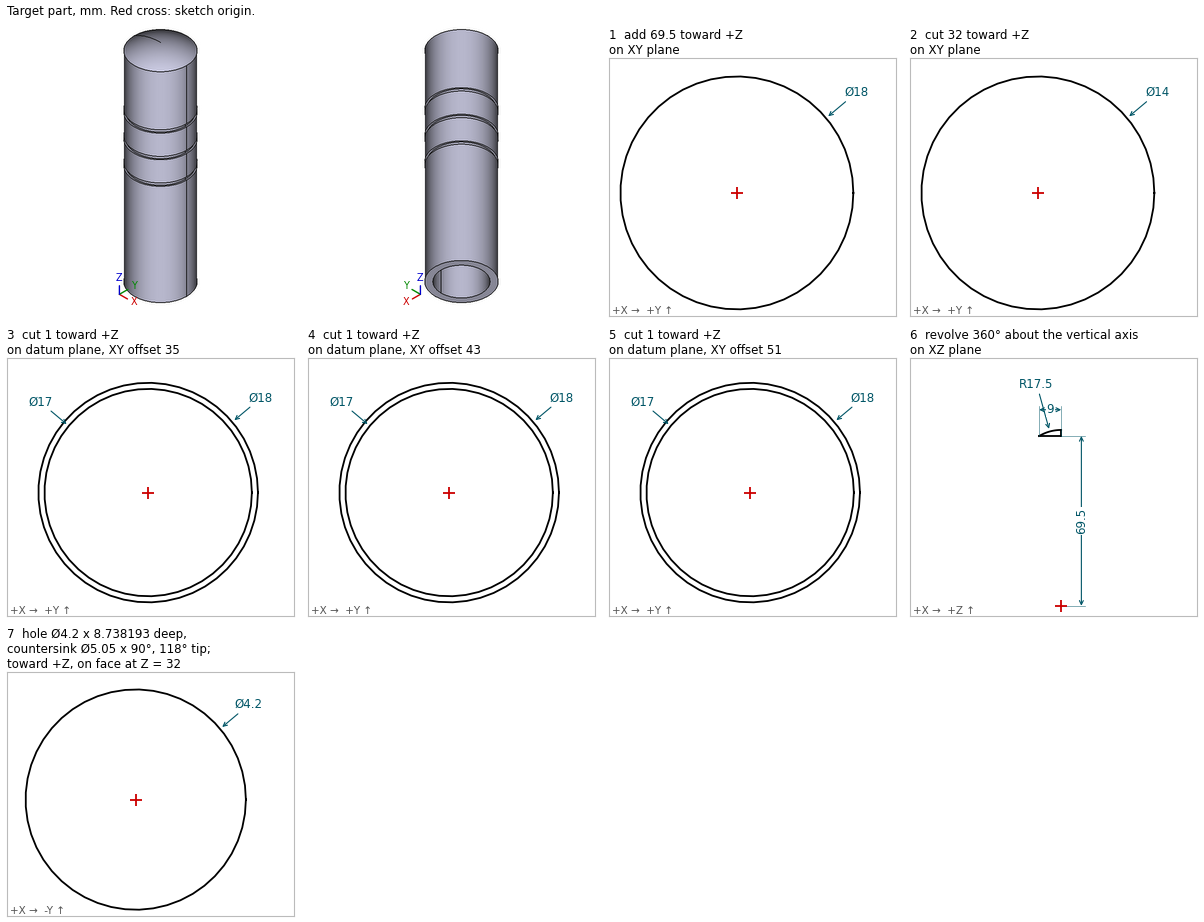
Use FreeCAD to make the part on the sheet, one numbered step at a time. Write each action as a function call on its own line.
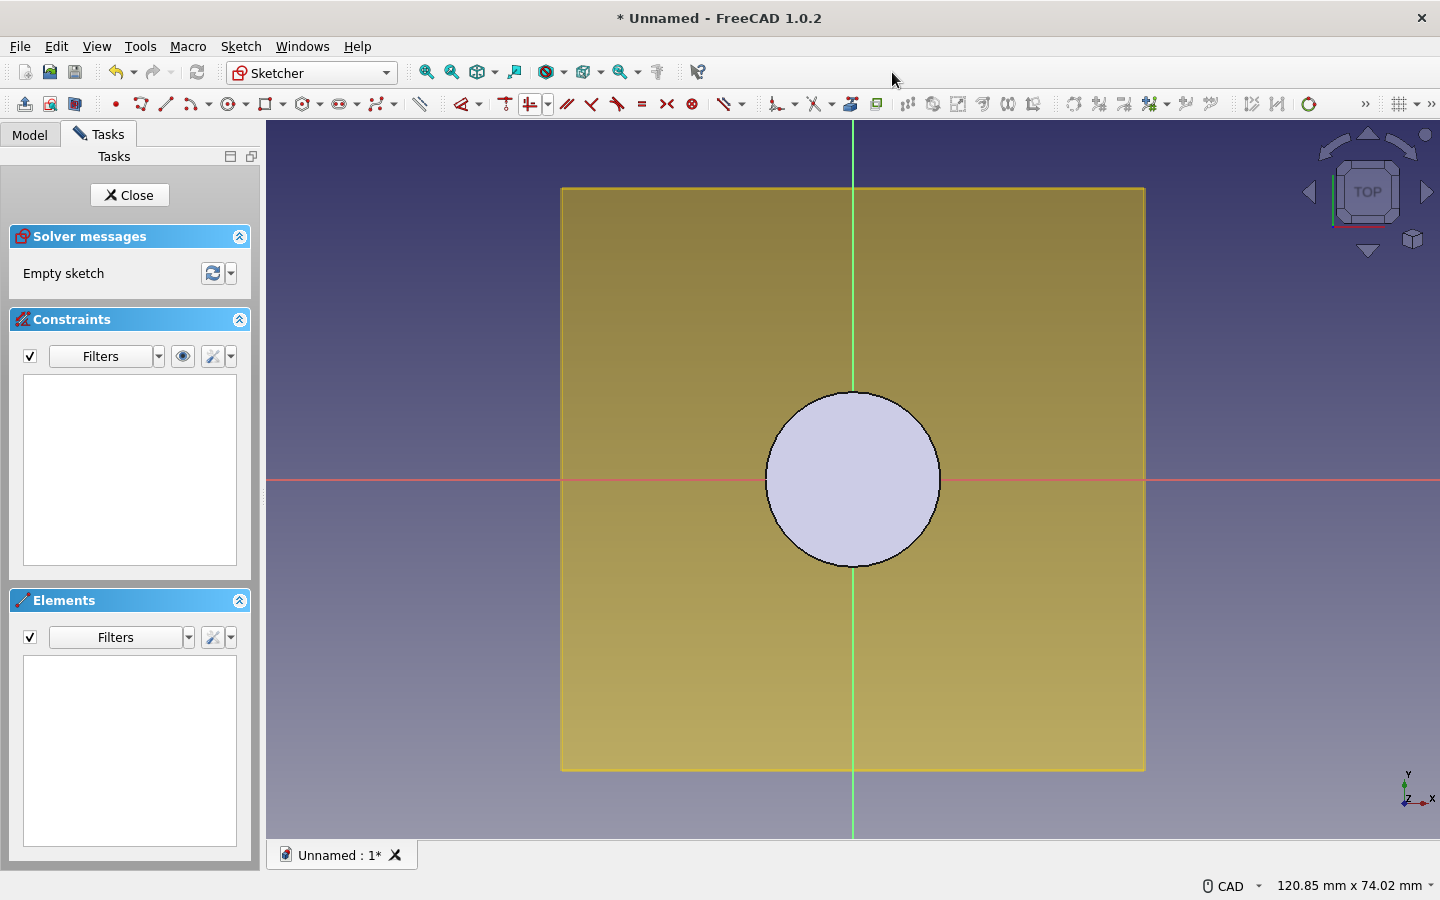
key(q)
key(s)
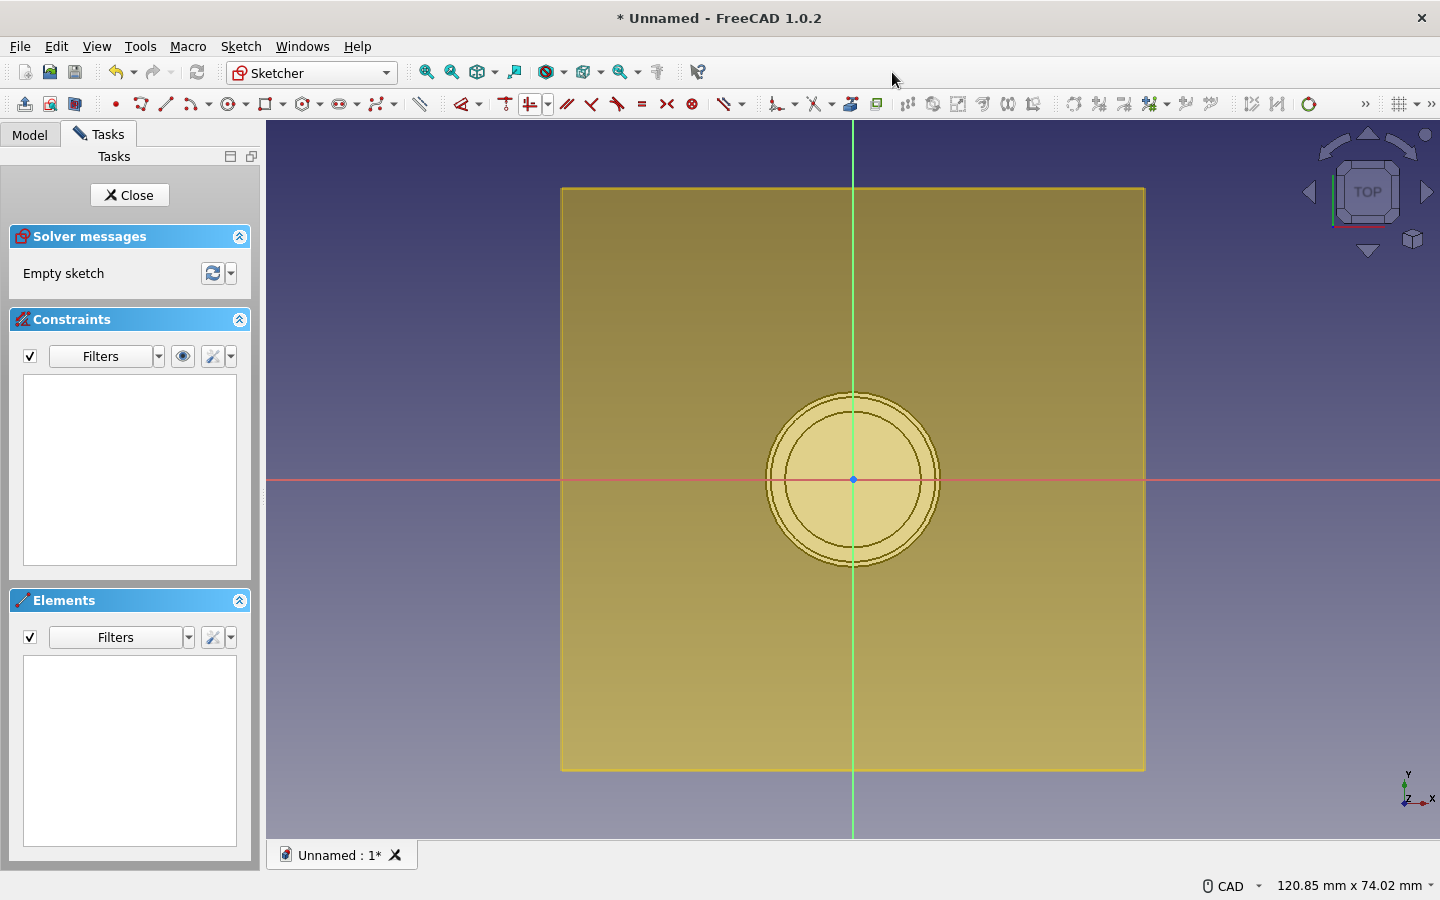
scroll(893, 480, up, 5)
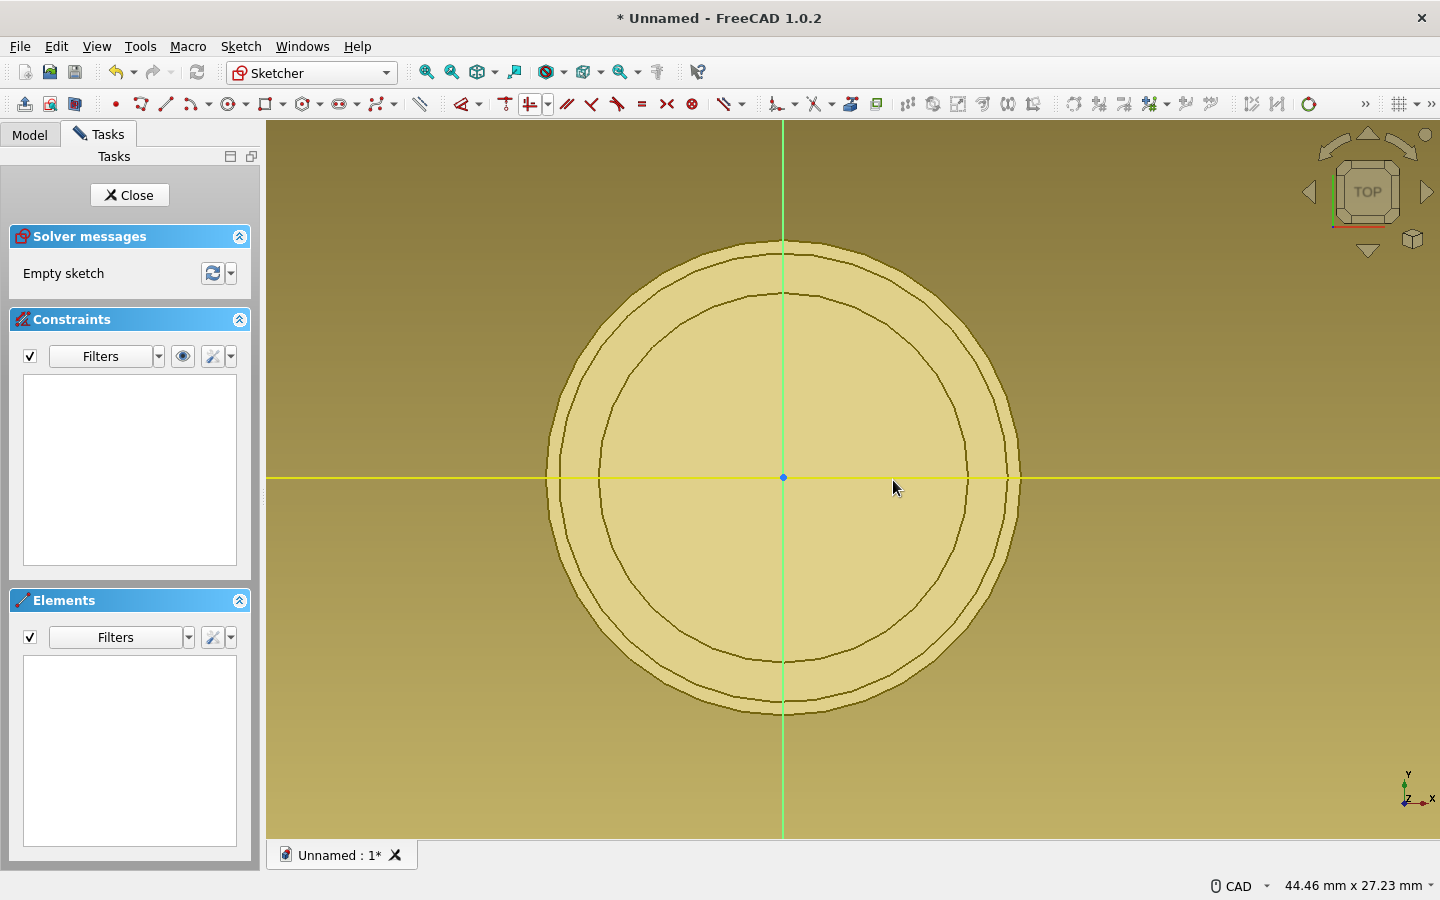
click(228, 104)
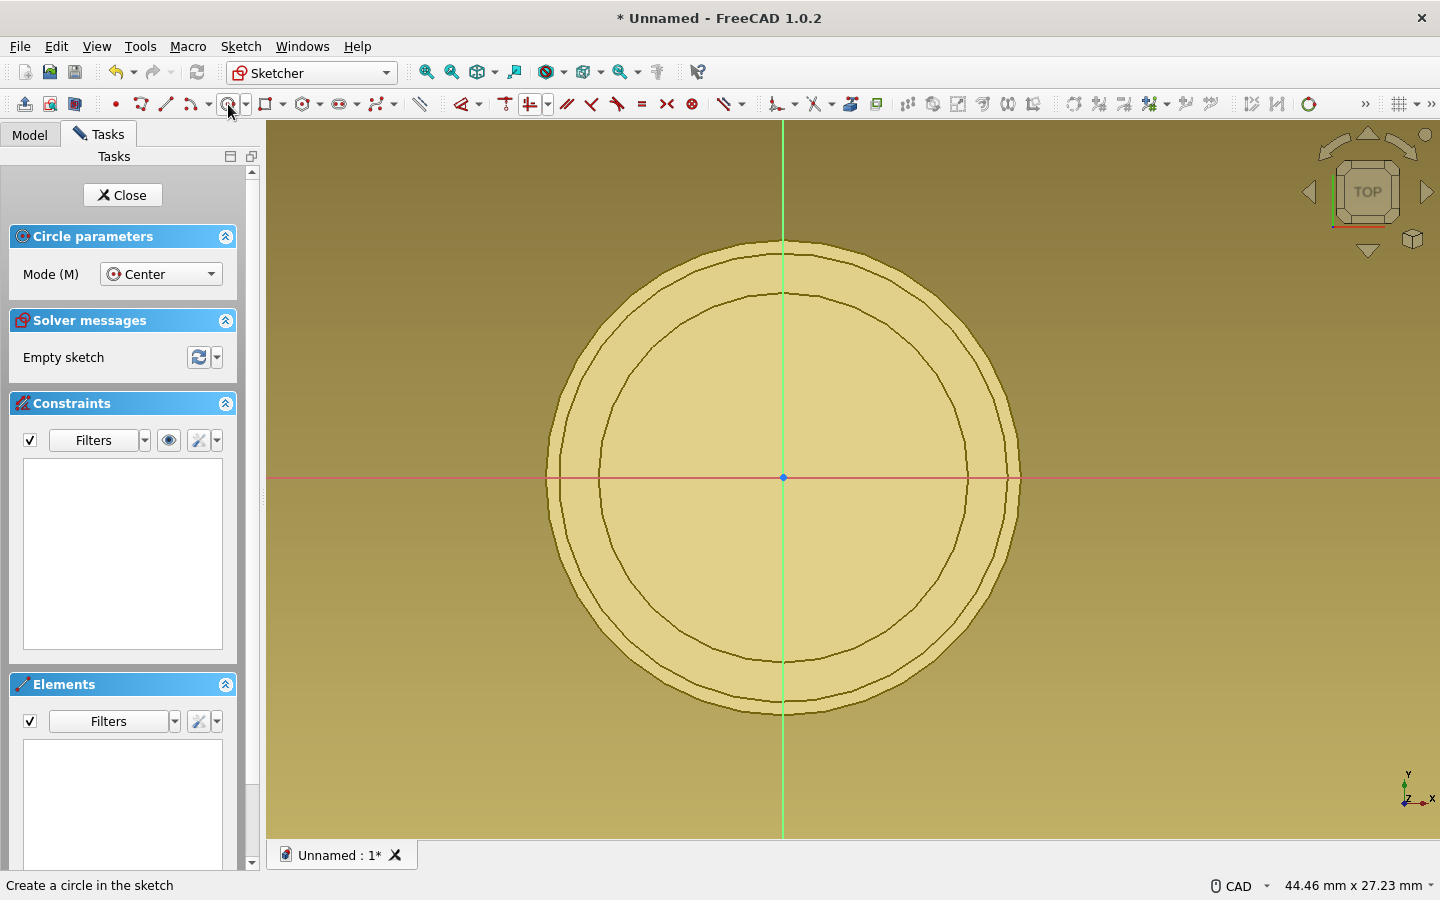
click(783, 478)
click(951, 310)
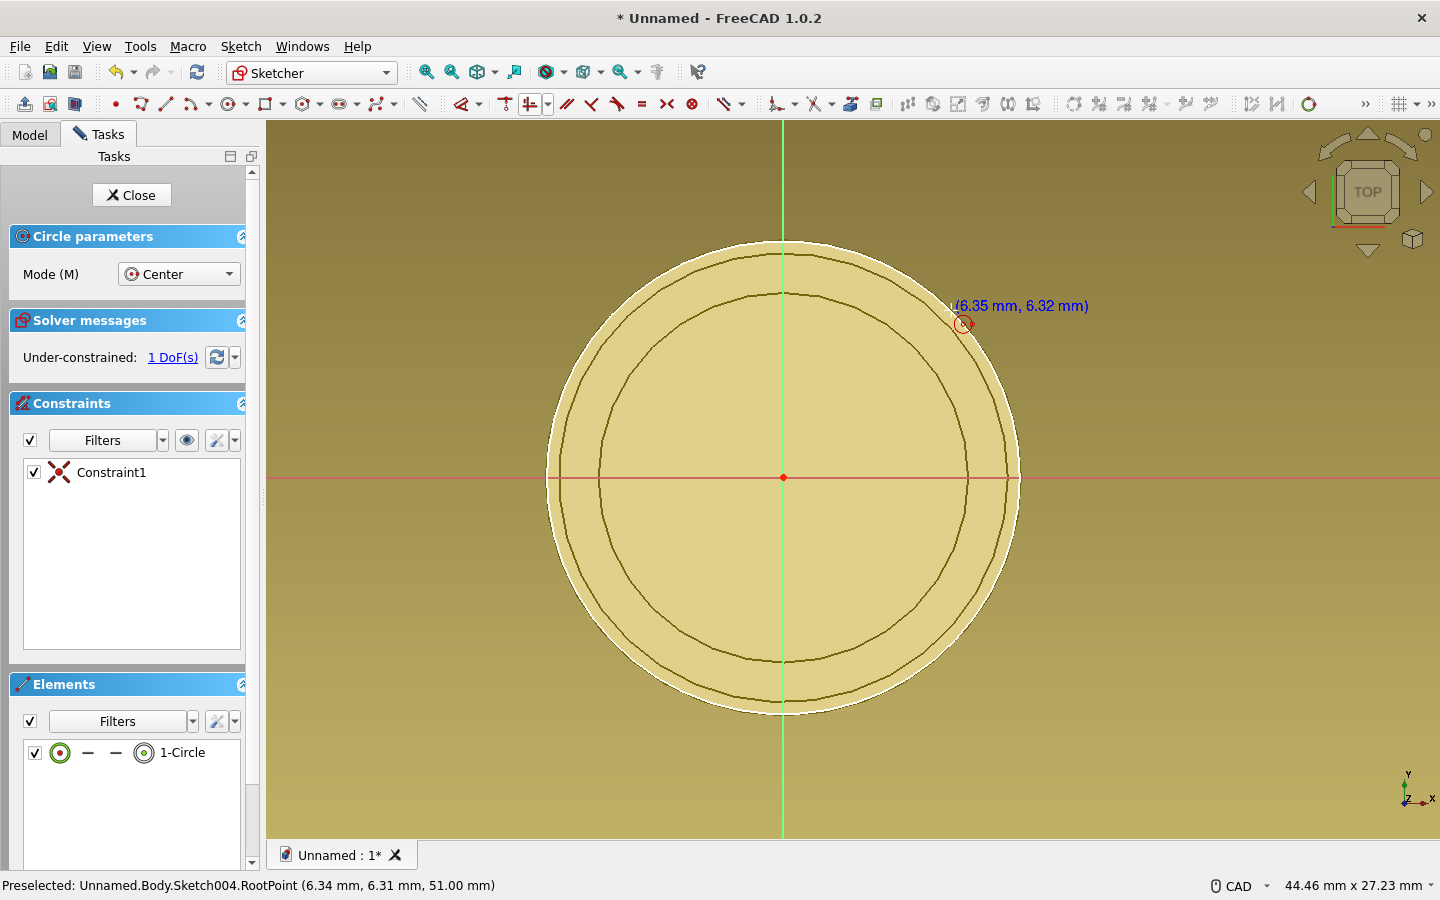
click(783, 478)
click(942, 319)
key(Escape)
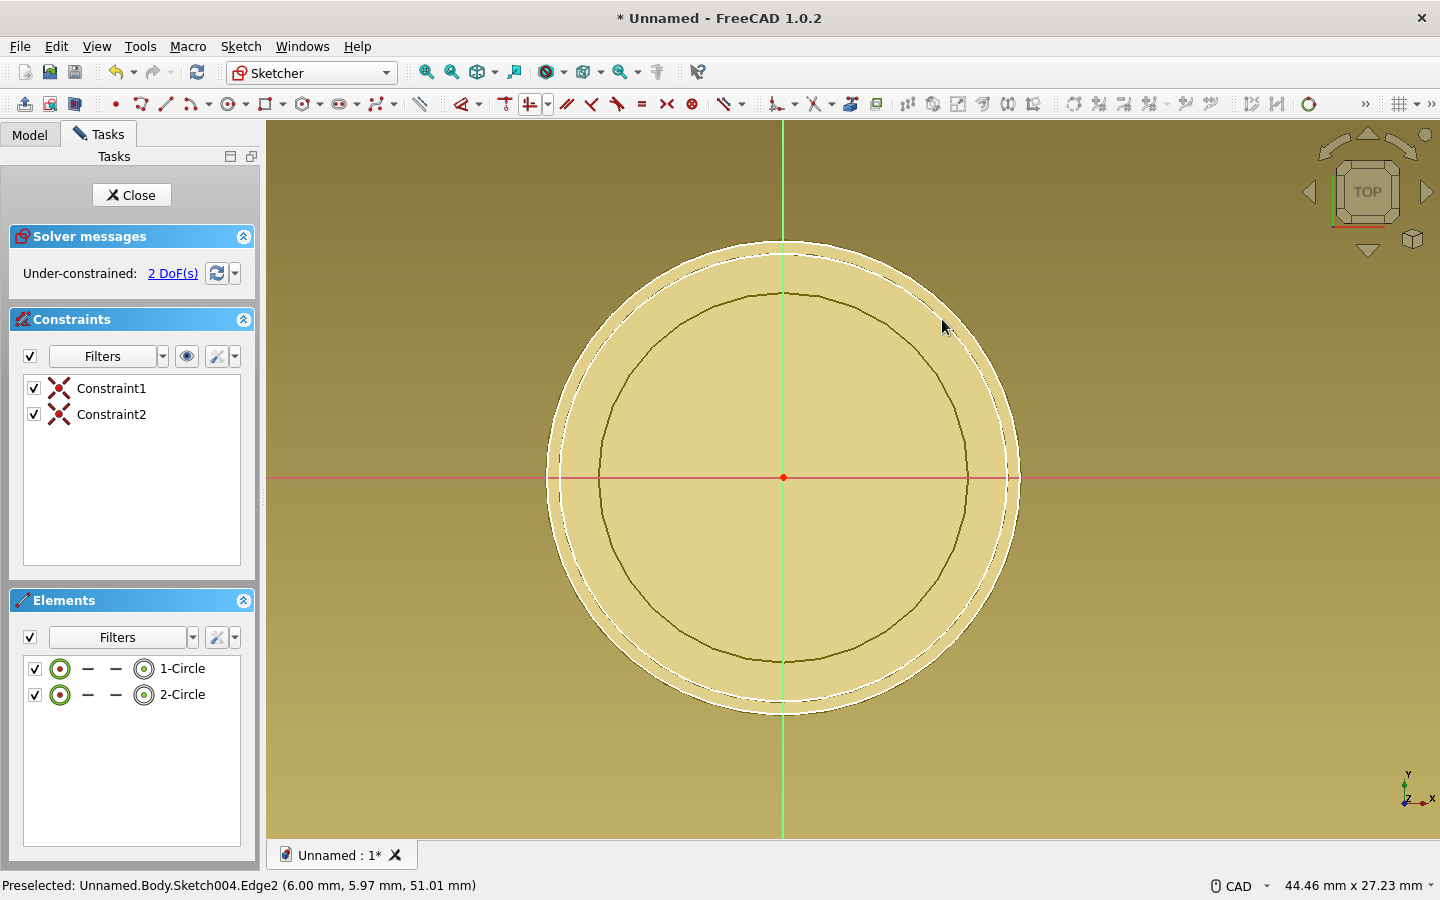
click(460, 104)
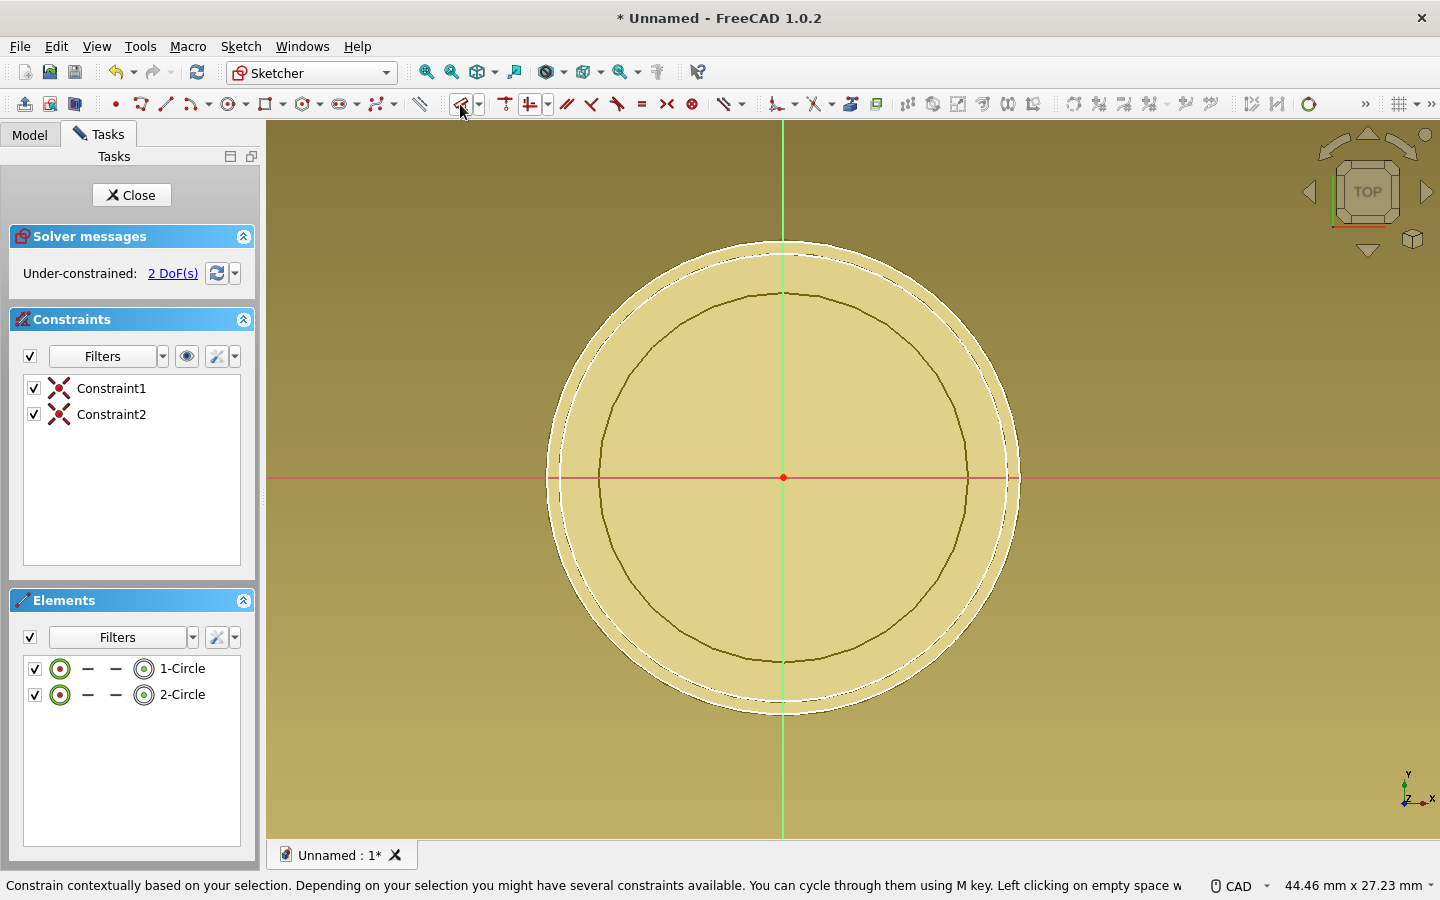
click(950, 310)
click(973, 287)